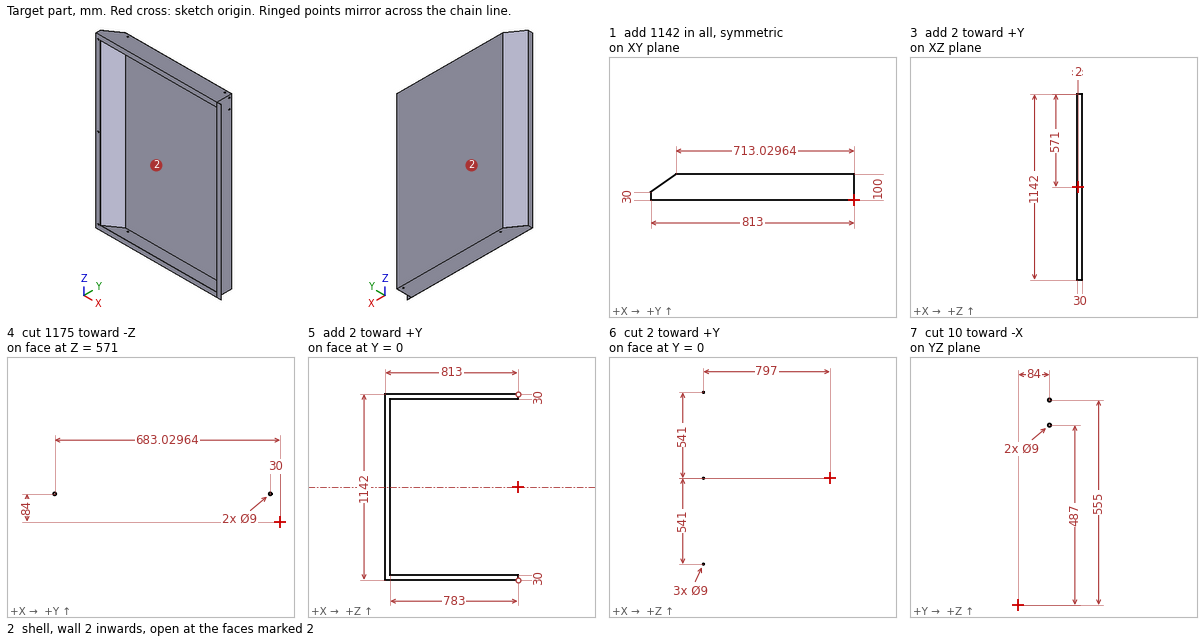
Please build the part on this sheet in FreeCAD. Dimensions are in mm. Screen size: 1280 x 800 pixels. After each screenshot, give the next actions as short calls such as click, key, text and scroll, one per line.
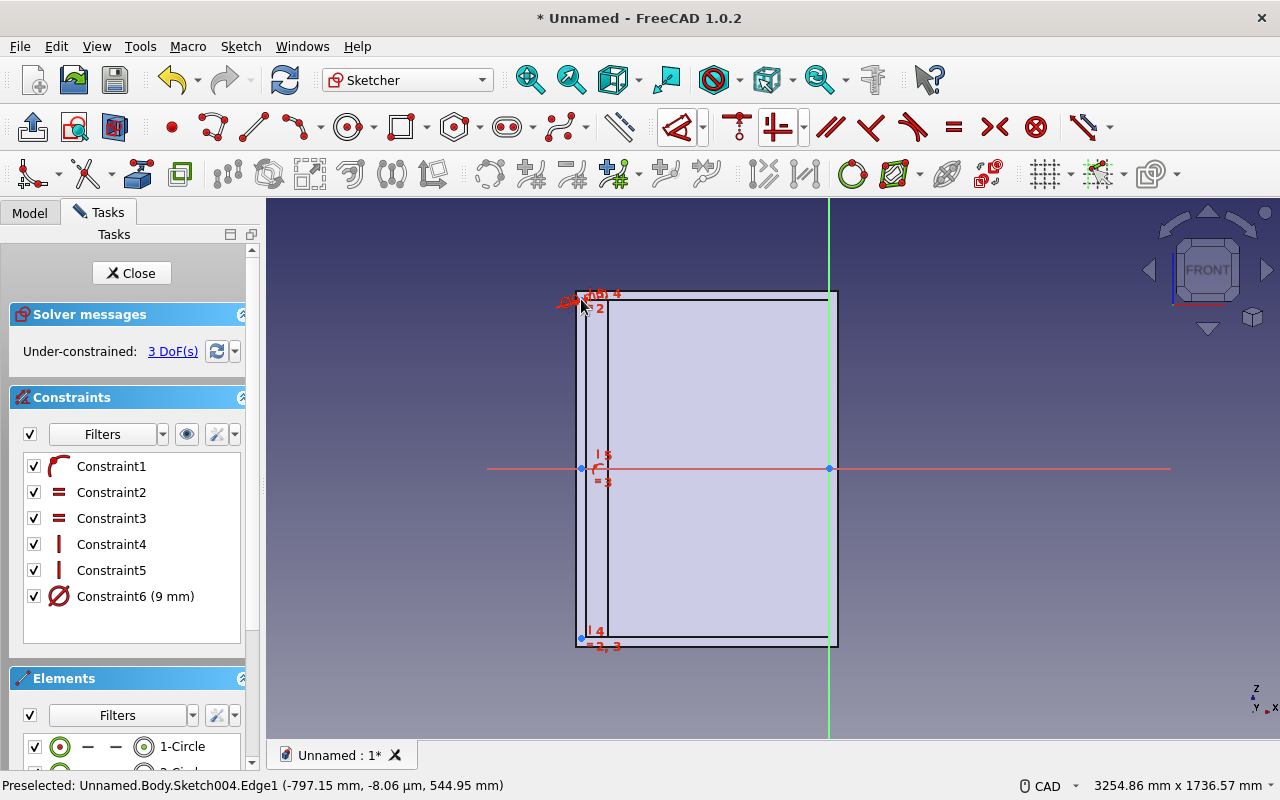
click(581, 301)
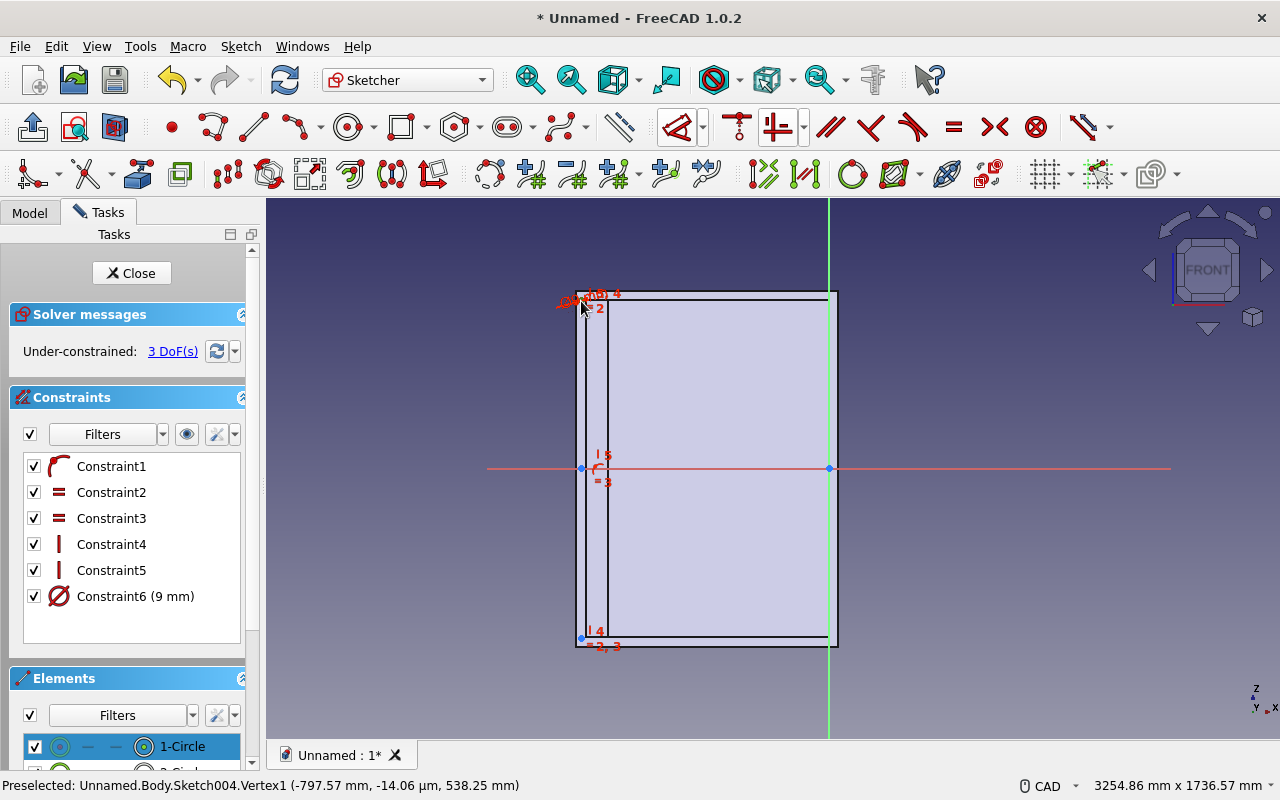
click(702, 128)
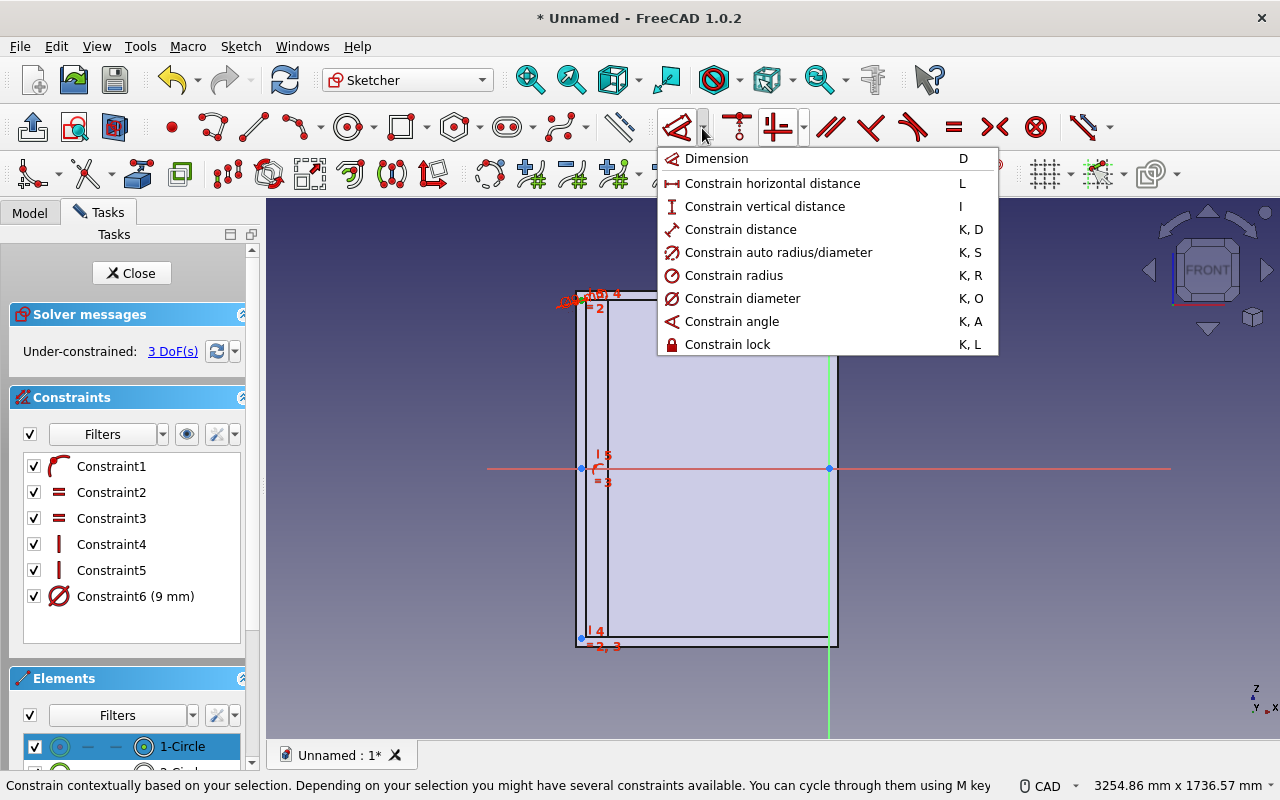
click(828, 184)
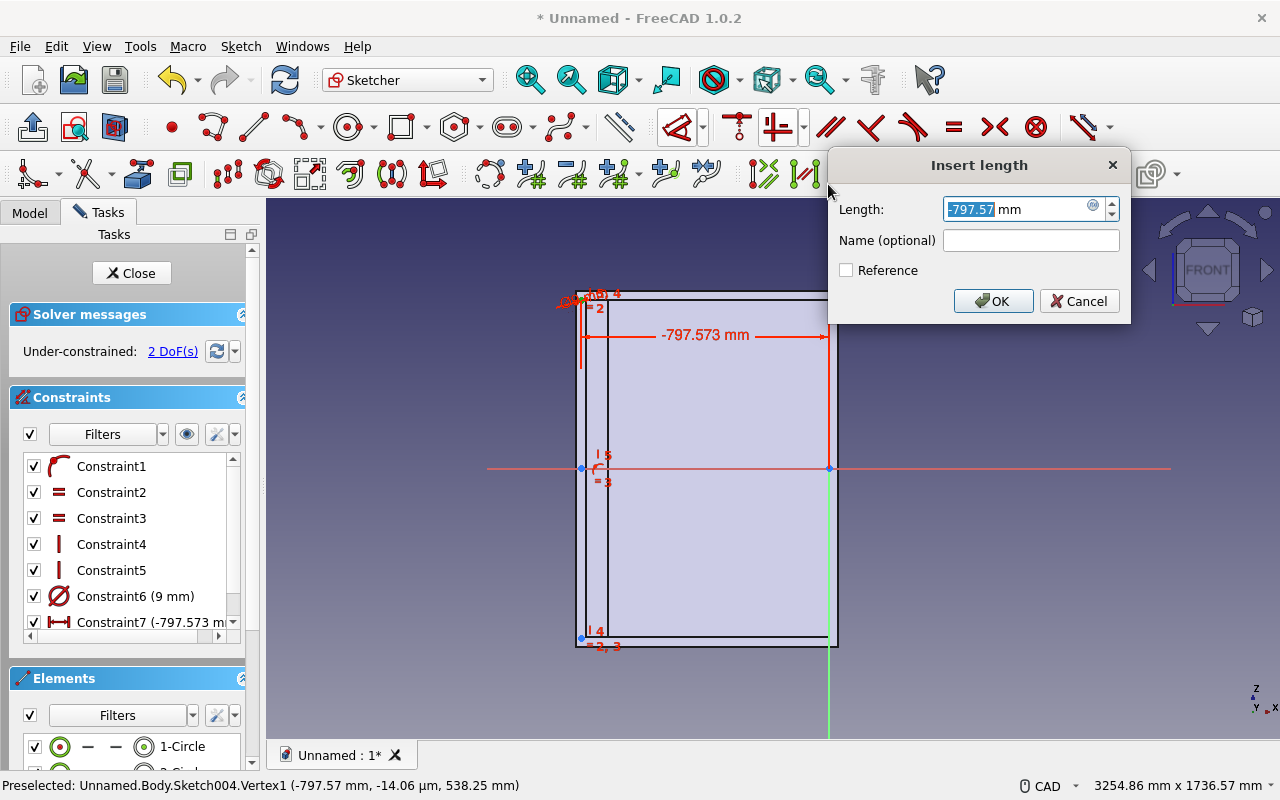
text(-797)
key(Return)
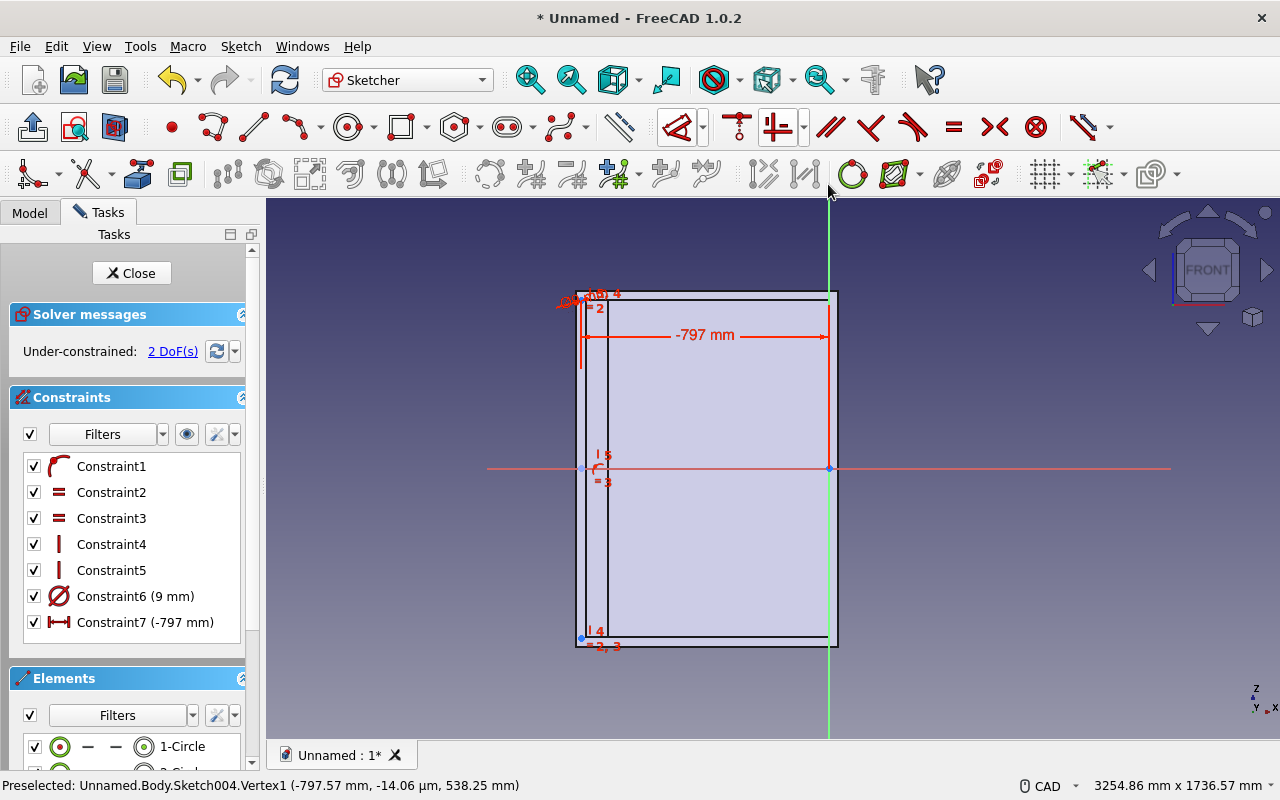
click(581, 301)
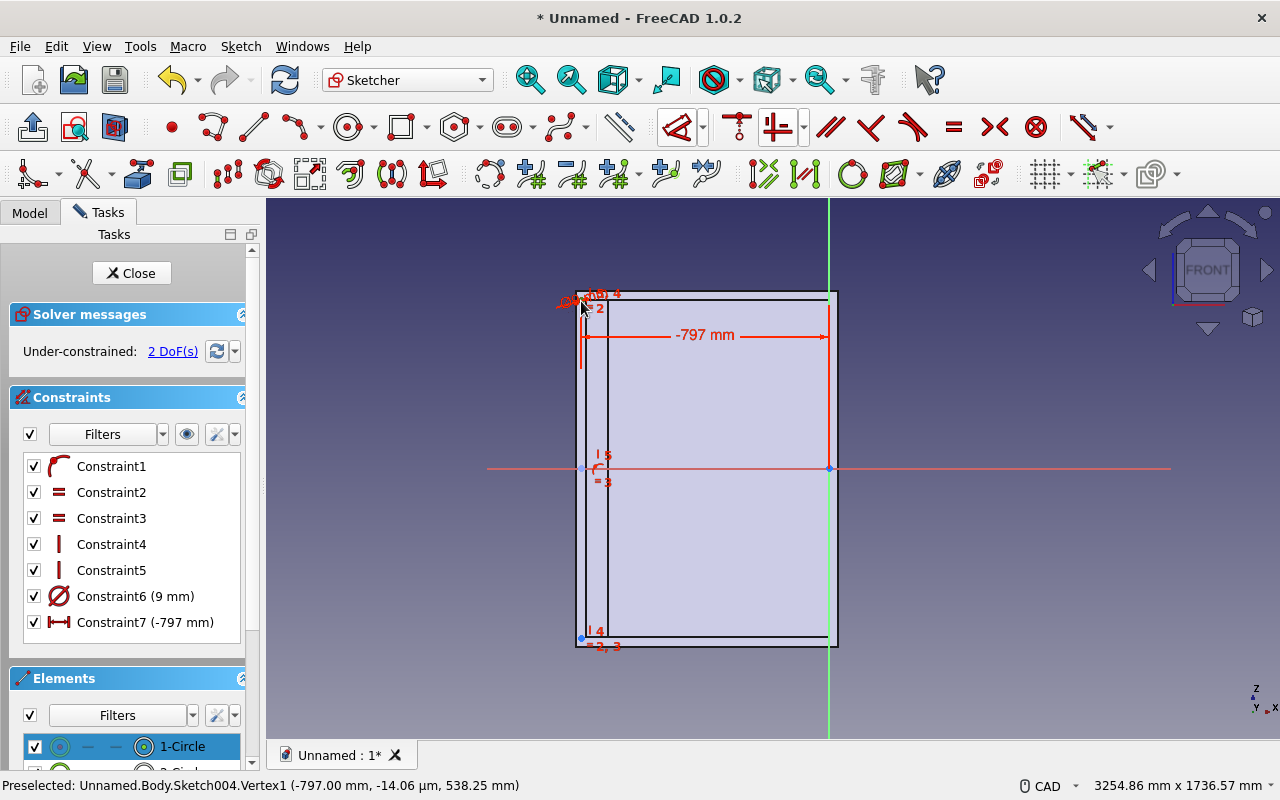
click(702, 128)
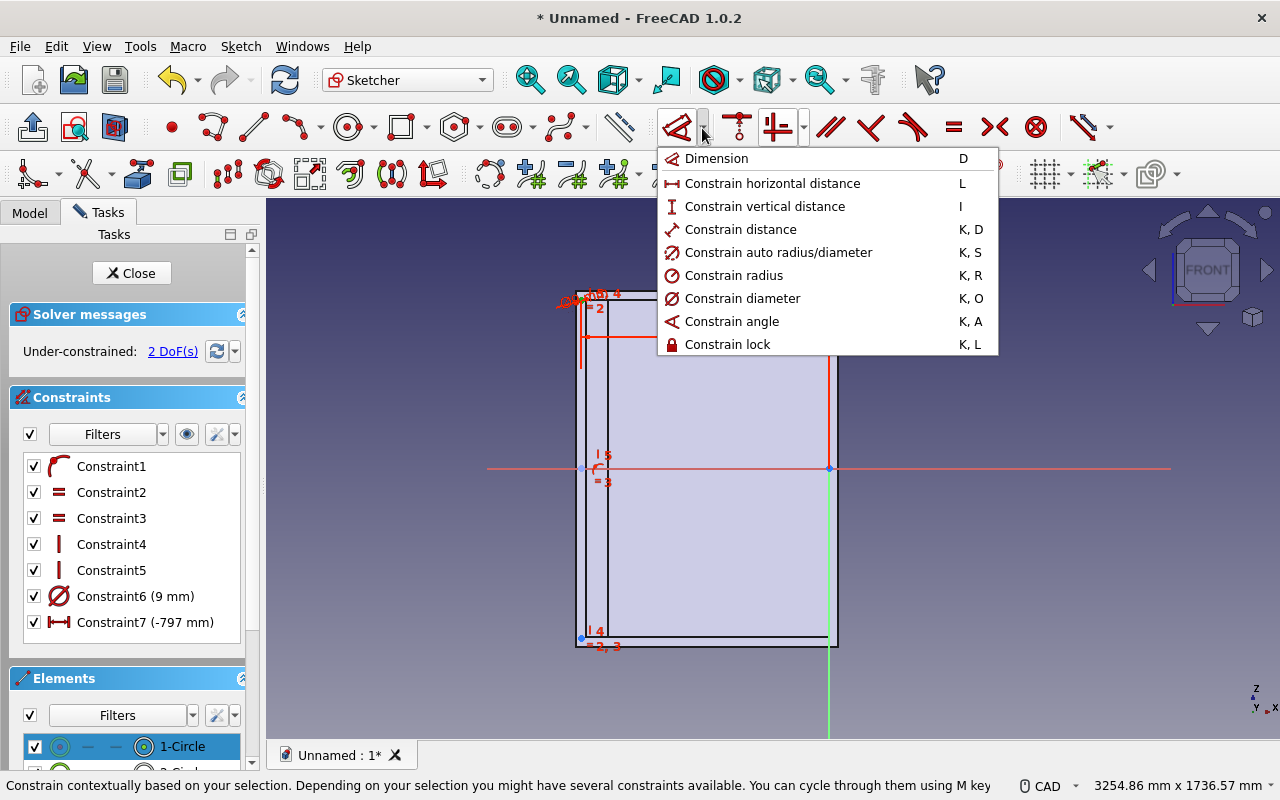
click(828, 206)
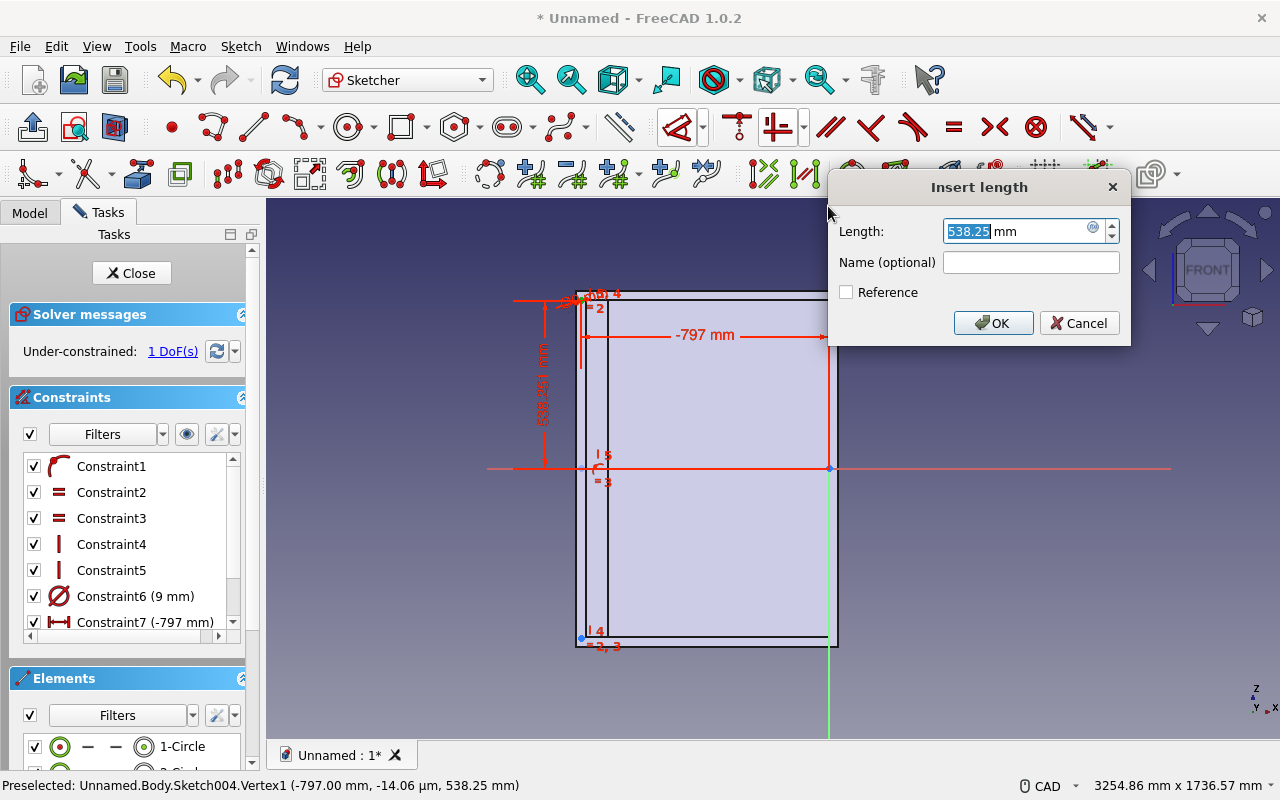
text(541)
key(Return)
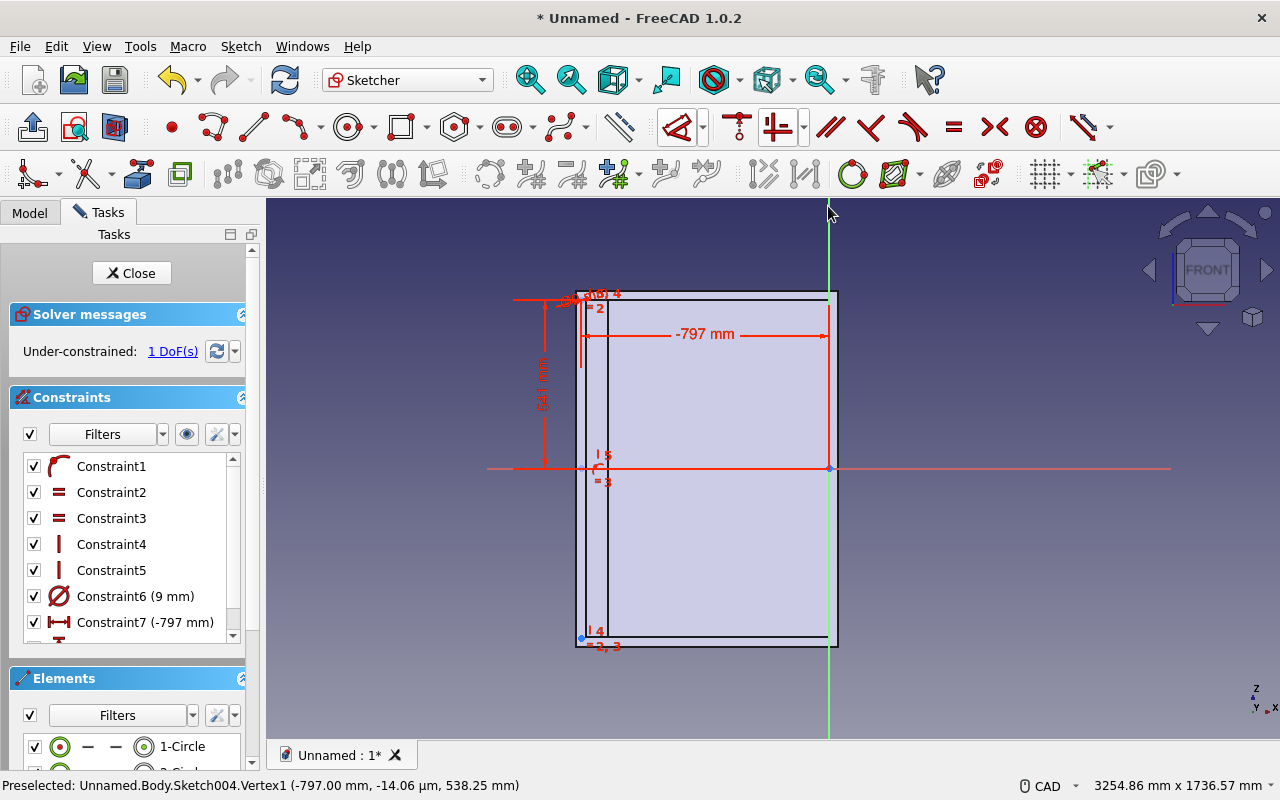
click(581, 638)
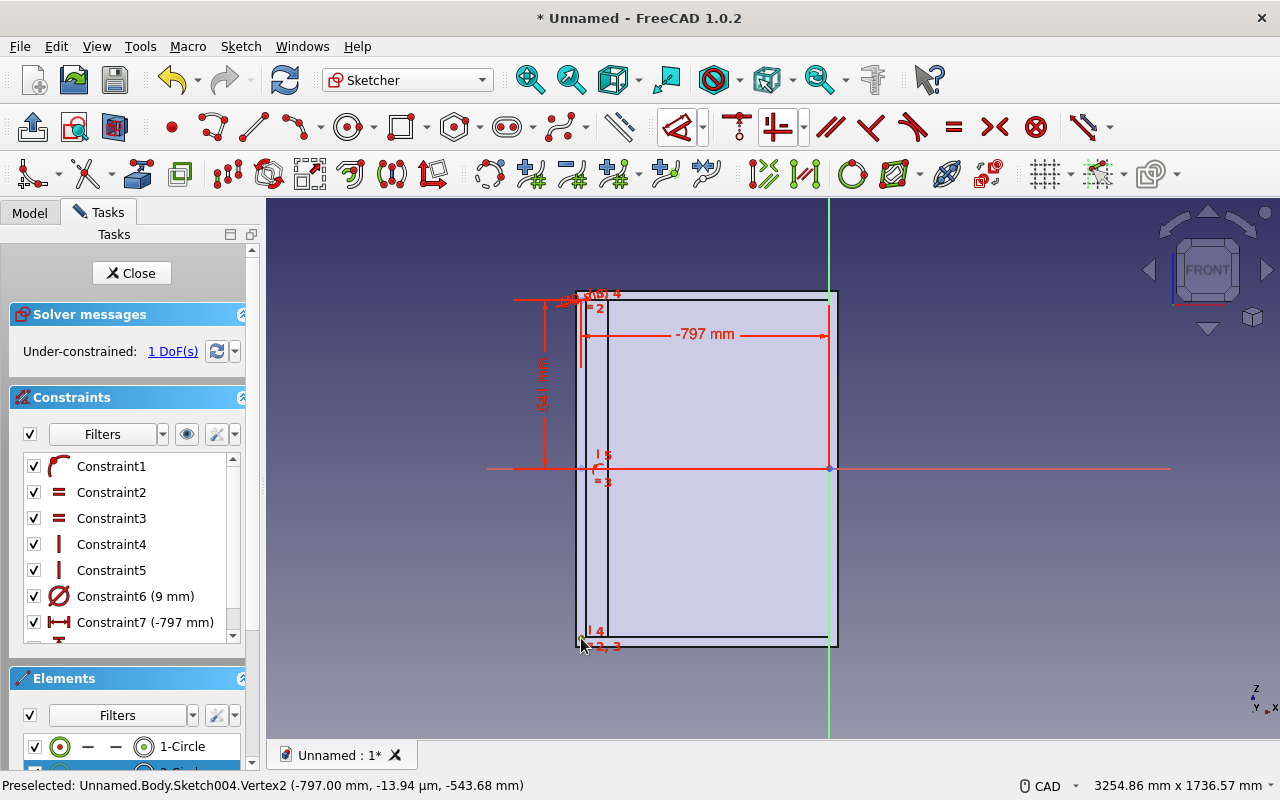
key(i)